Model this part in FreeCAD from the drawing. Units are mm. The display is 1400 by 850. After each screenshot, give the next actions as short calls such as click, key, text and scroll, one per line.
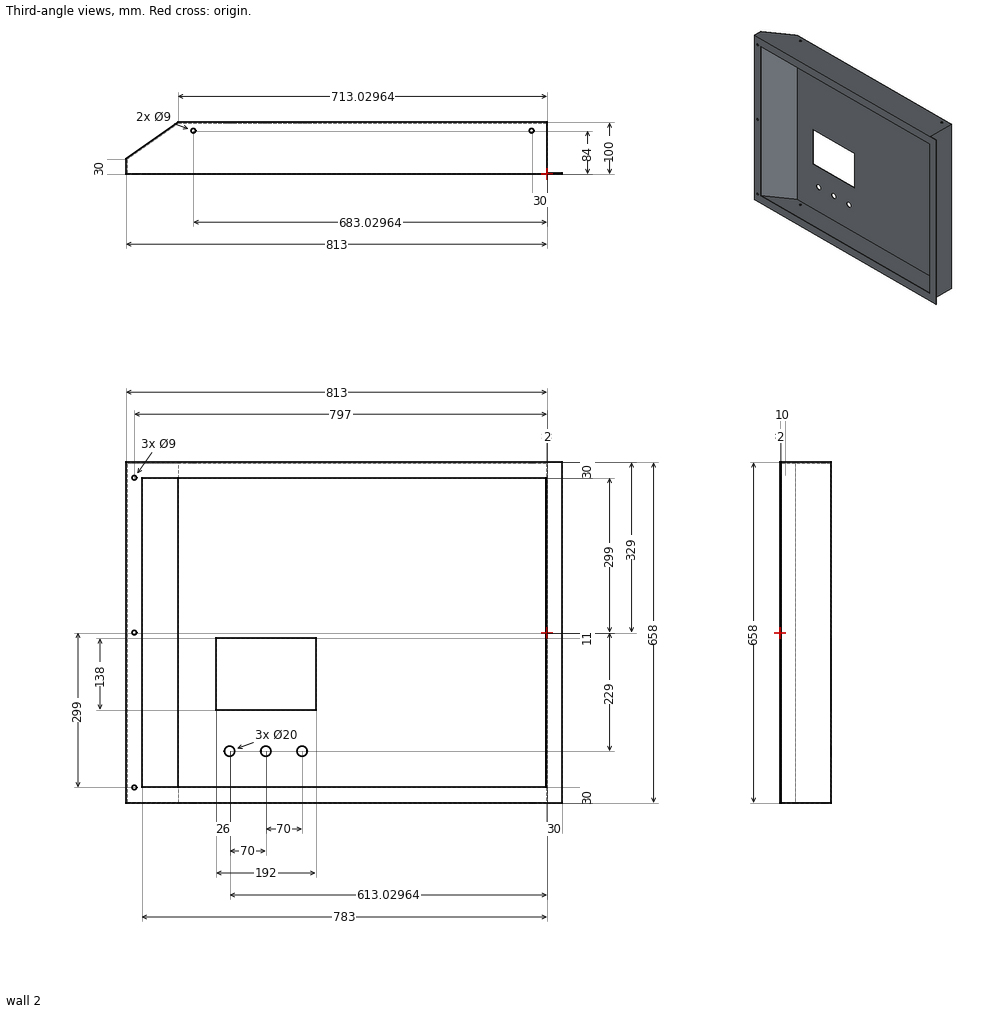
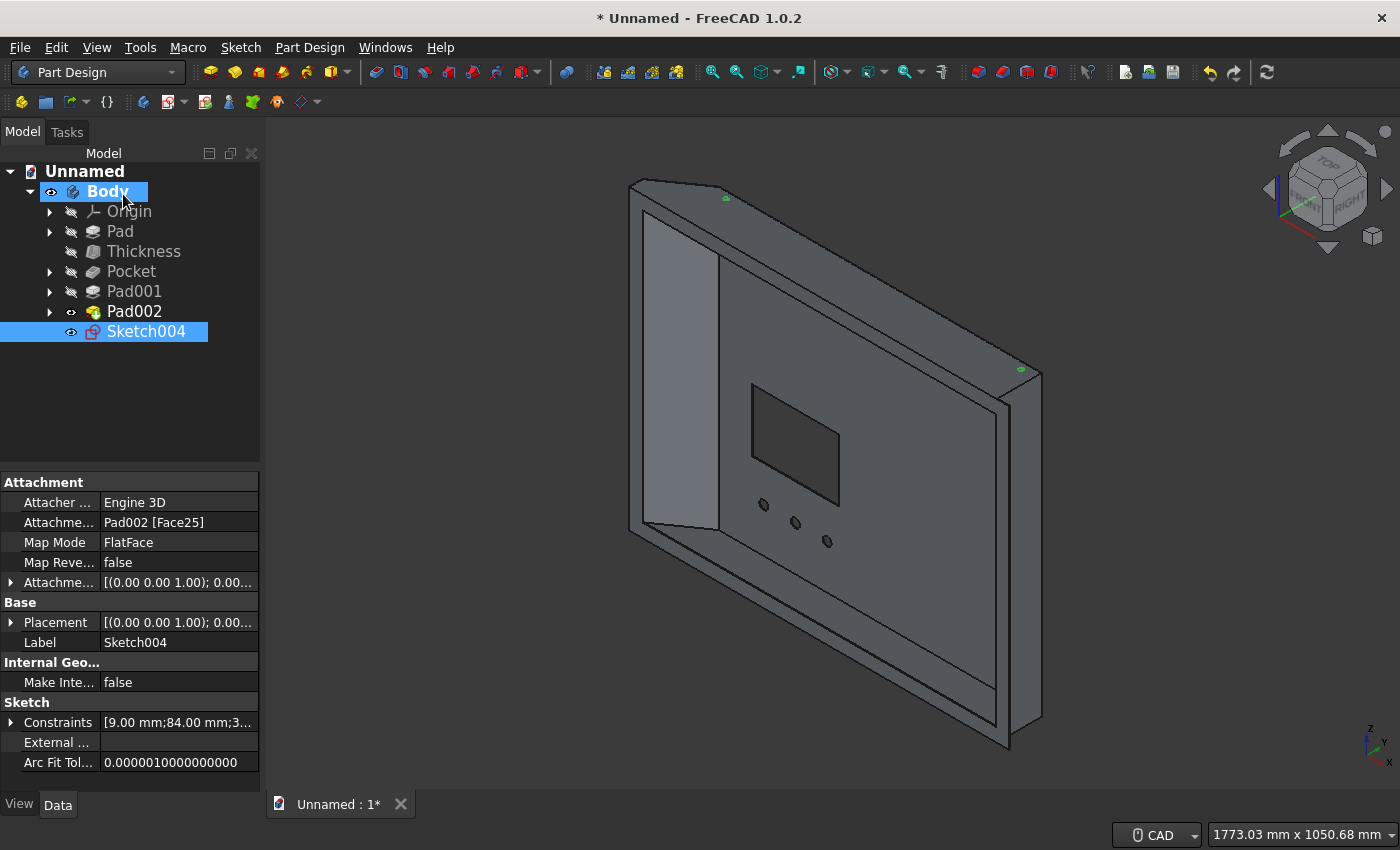
click(378, 72)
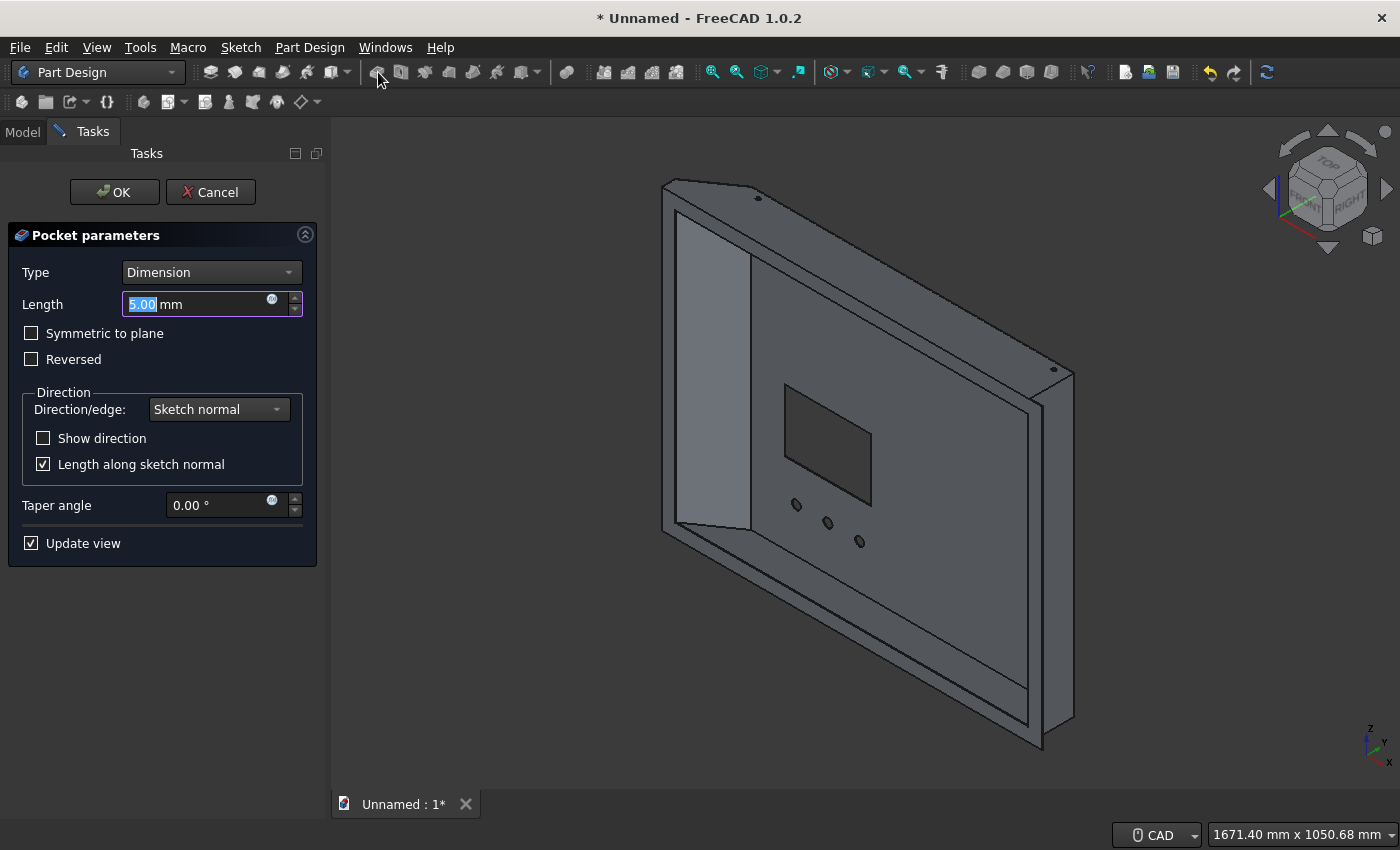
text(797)
key(Tab)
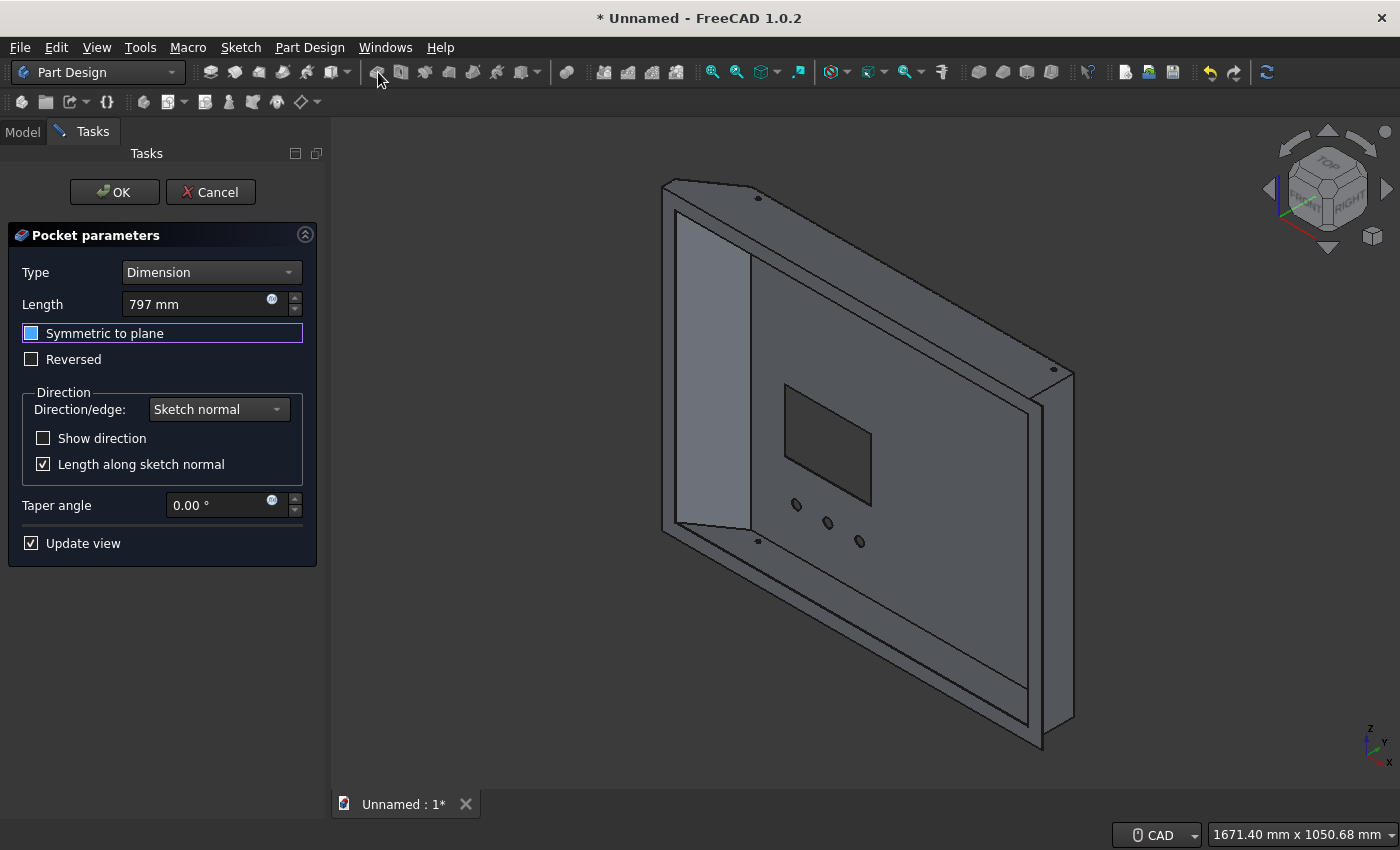
click(115, 192)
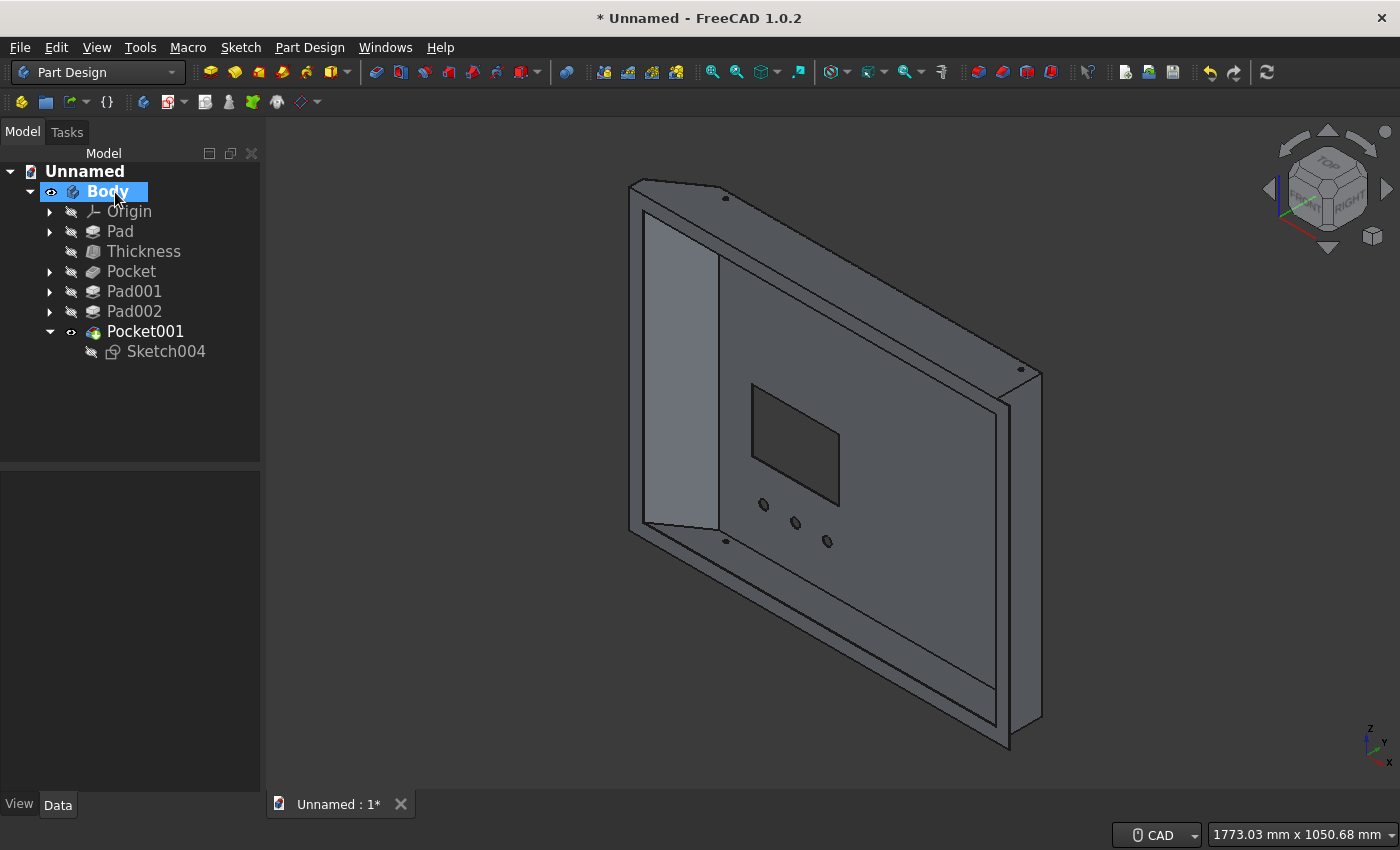
click(168, 102)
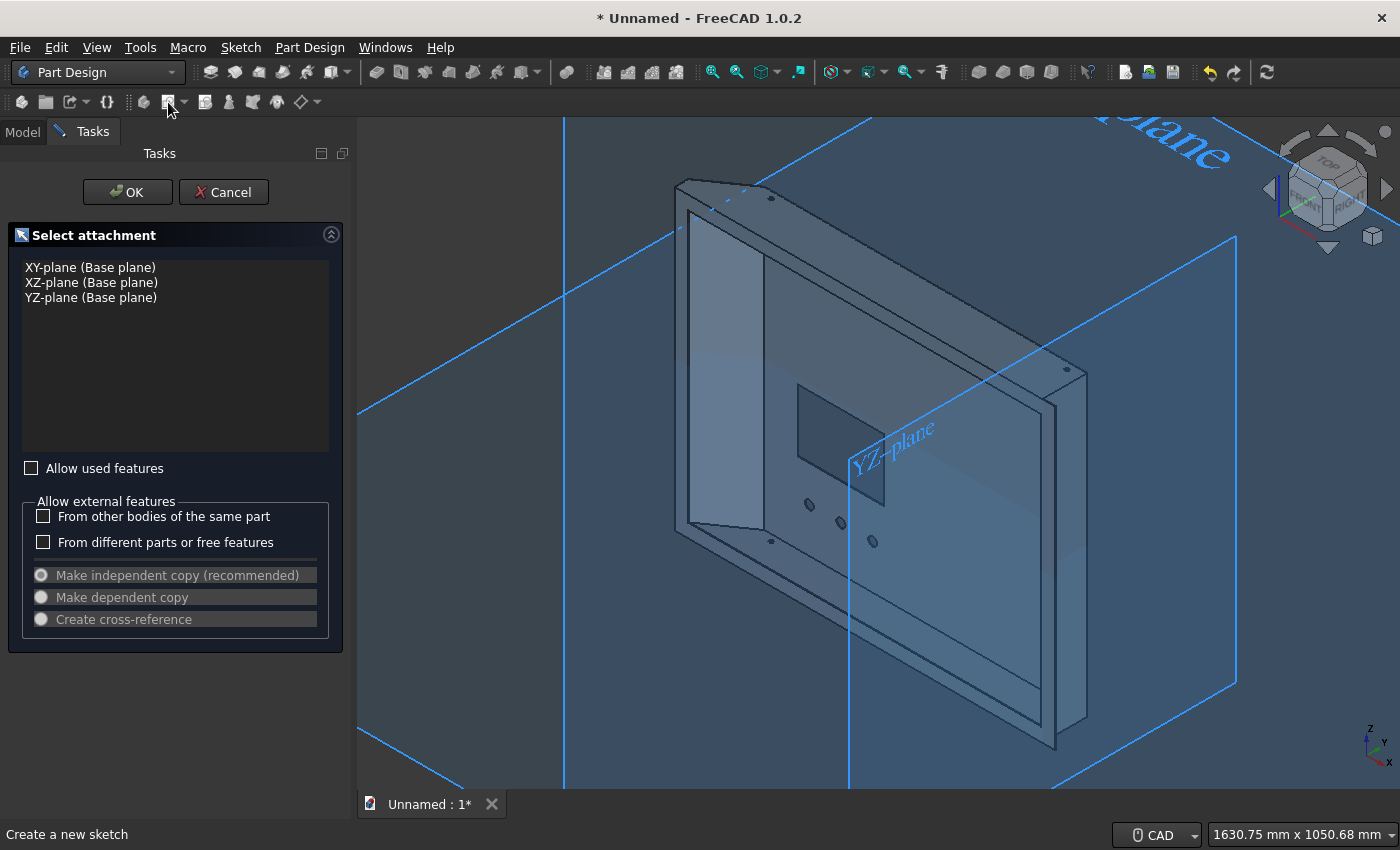
click(82, 282)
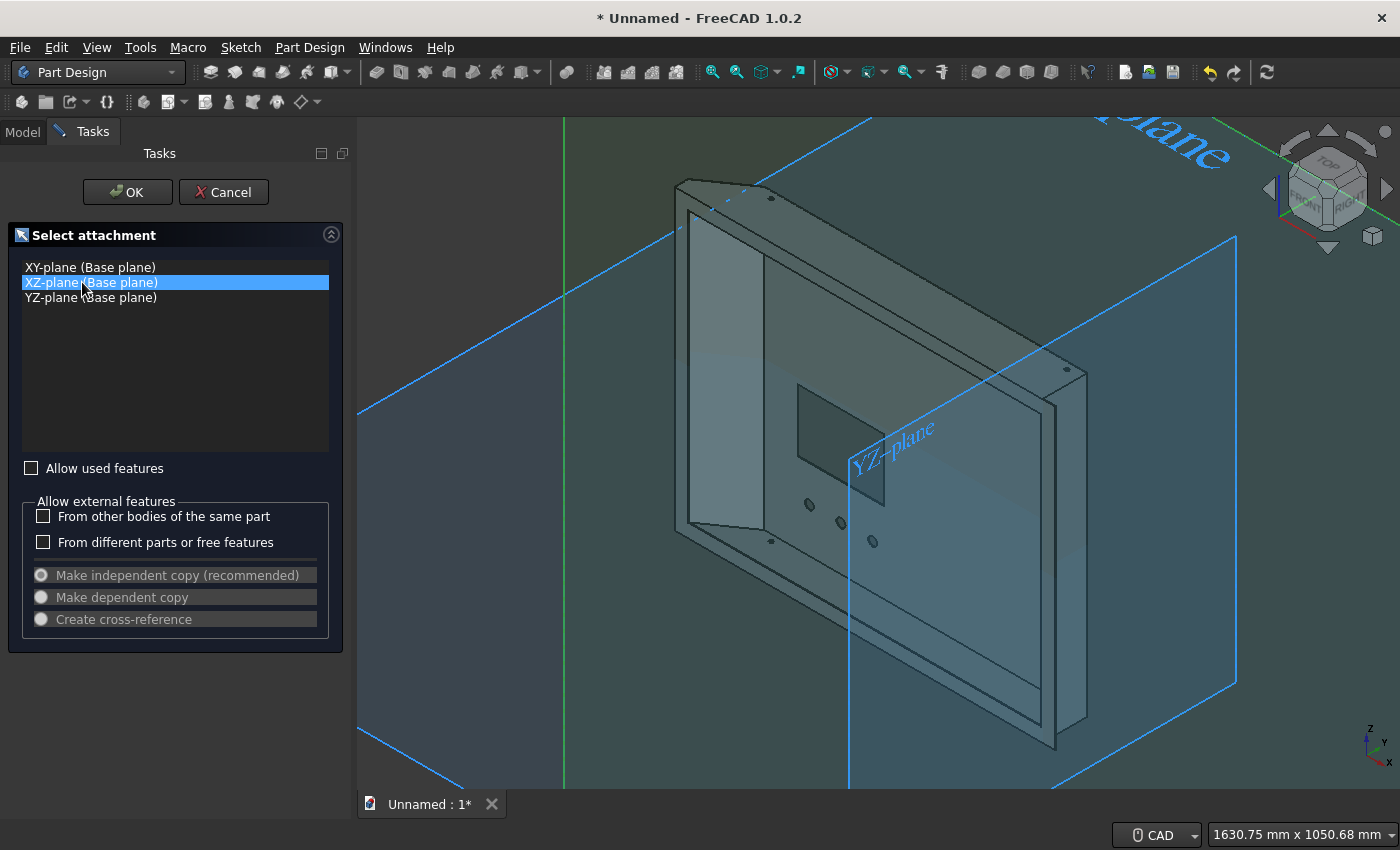
click(128, 192)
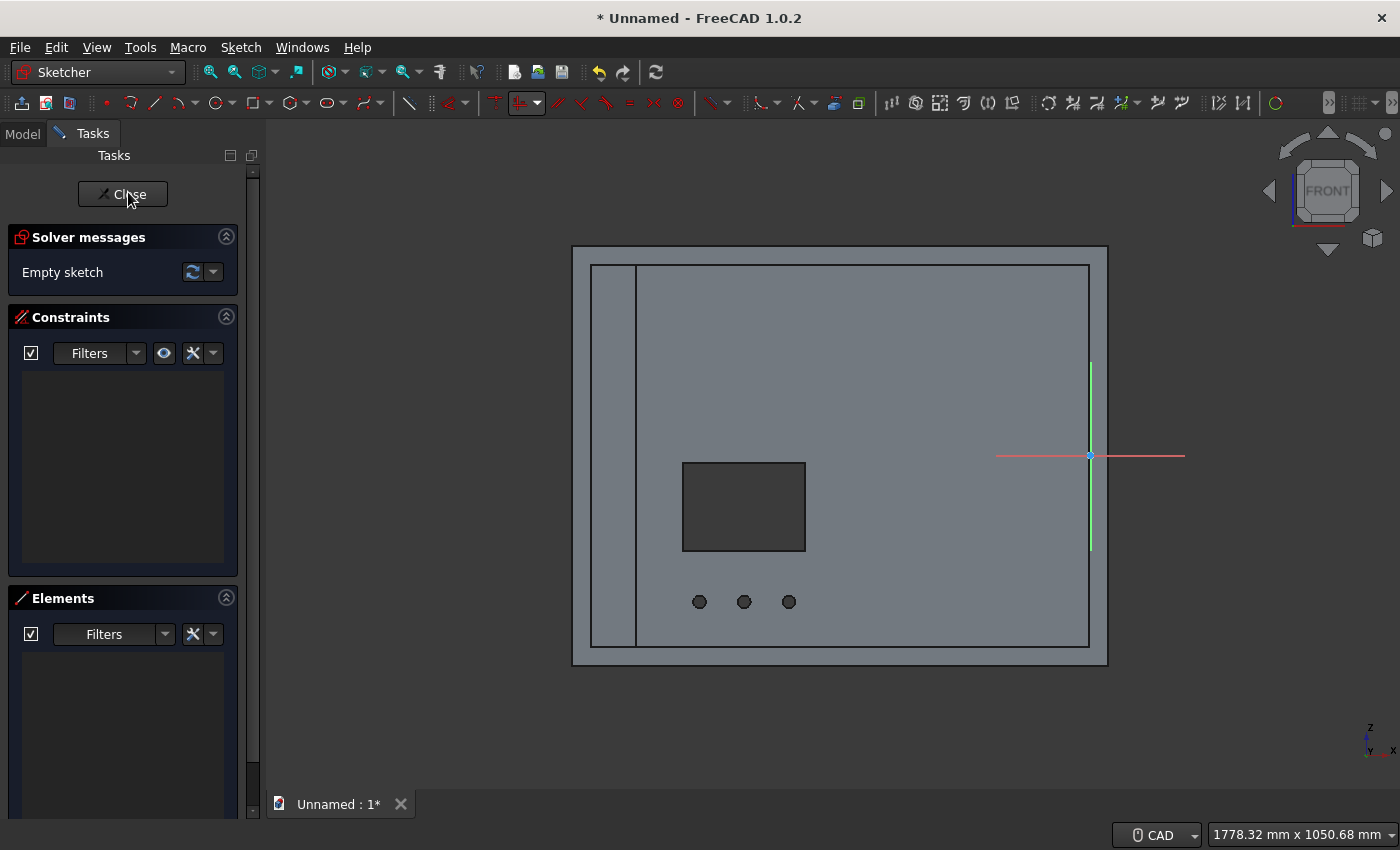
click(216, 104)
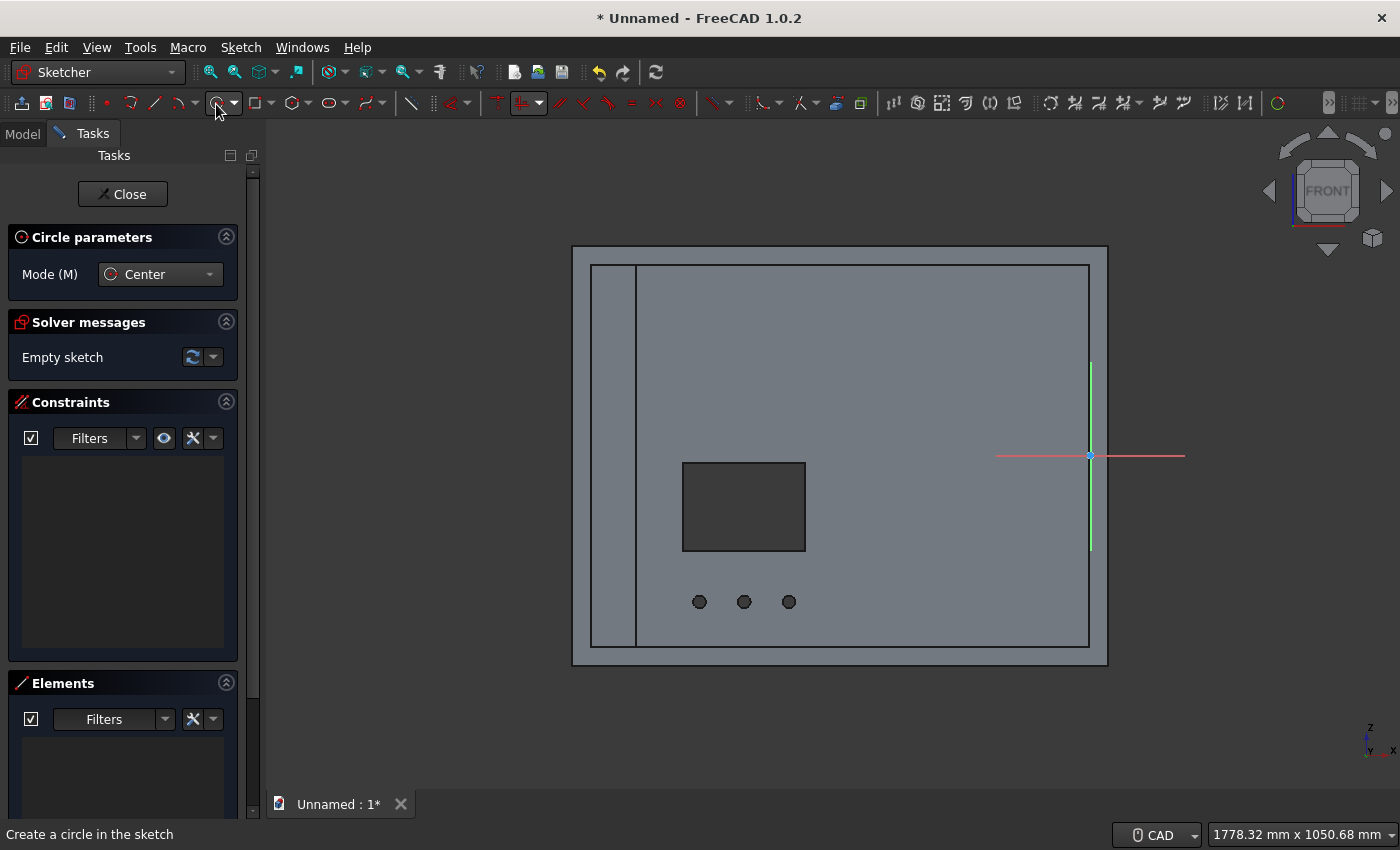
scroll(582, 265, up, 11)